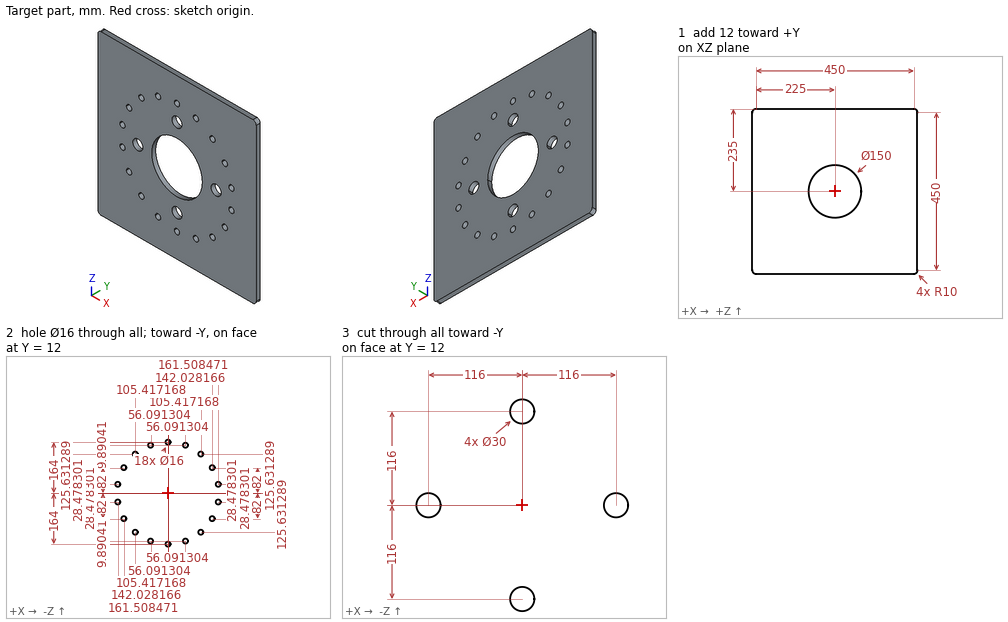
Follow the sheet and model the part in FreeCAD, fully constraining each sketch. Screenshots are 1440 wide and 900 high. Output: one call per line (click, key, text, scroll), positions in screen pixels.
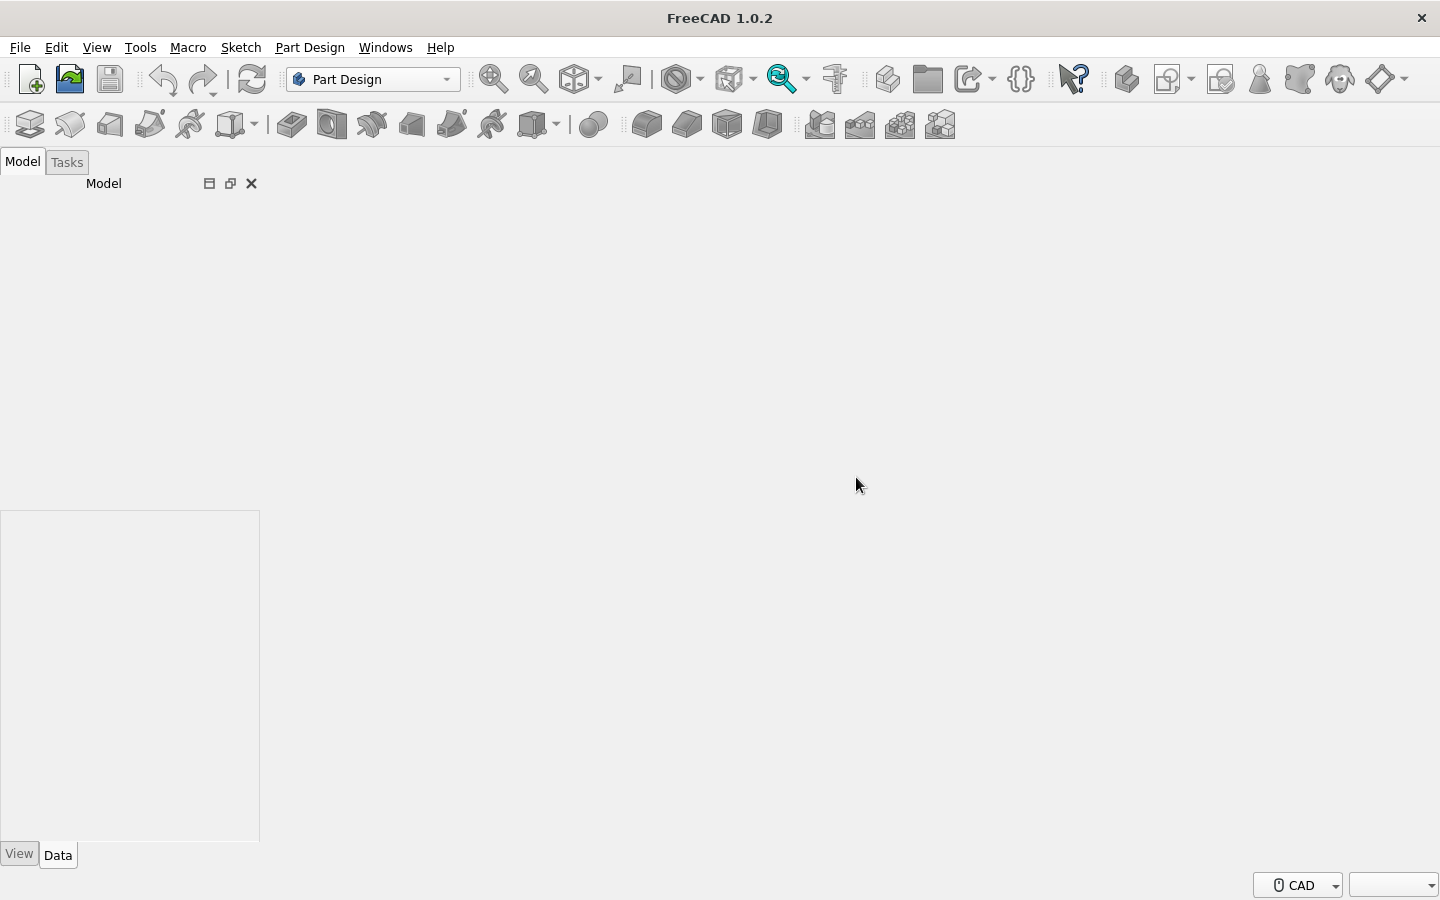
click(30, 80)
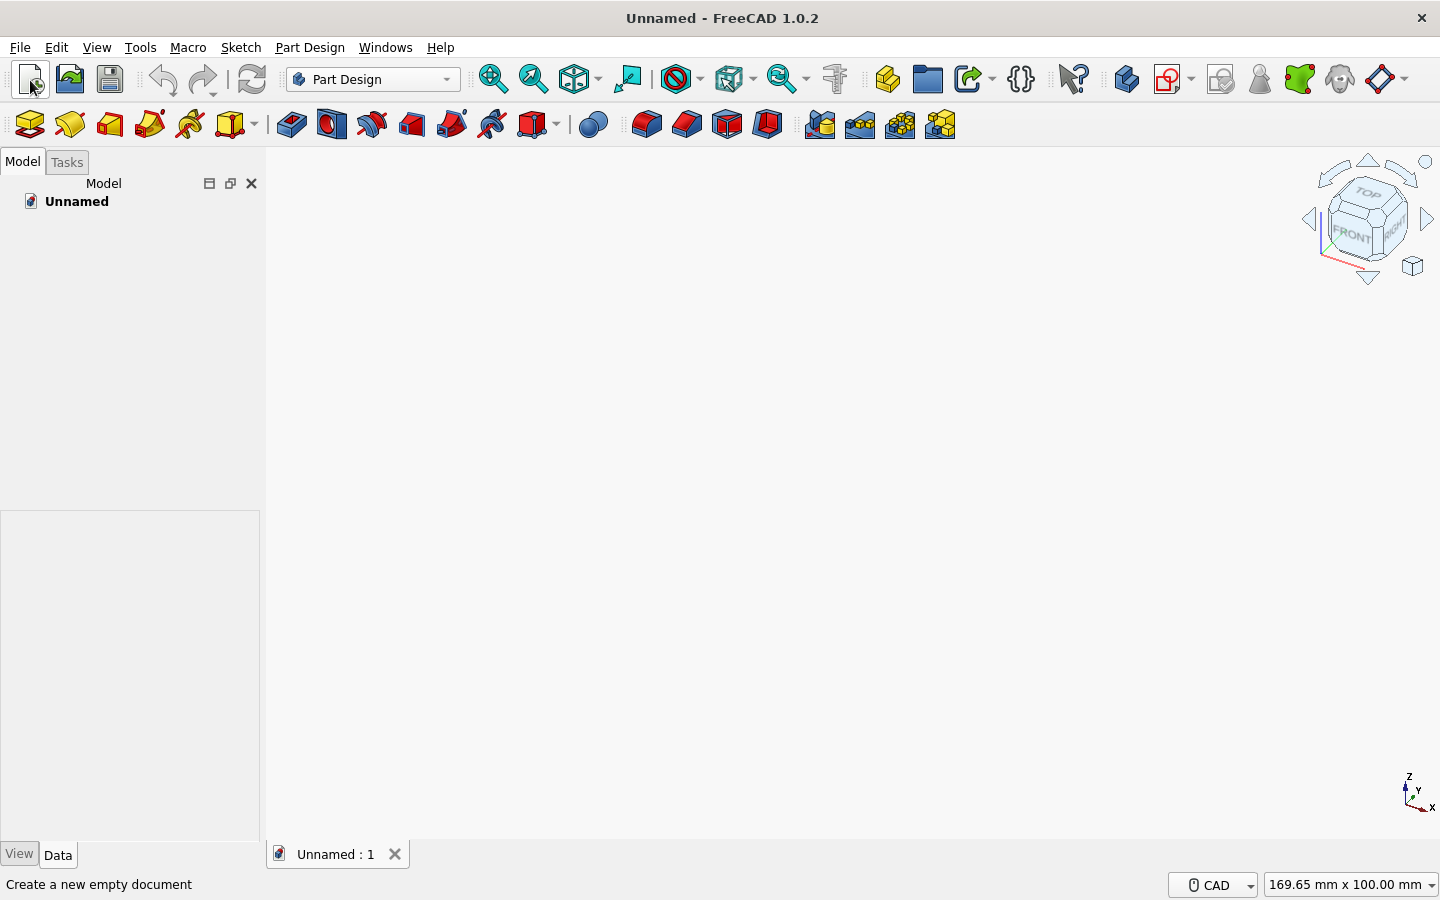
click(1168, 80)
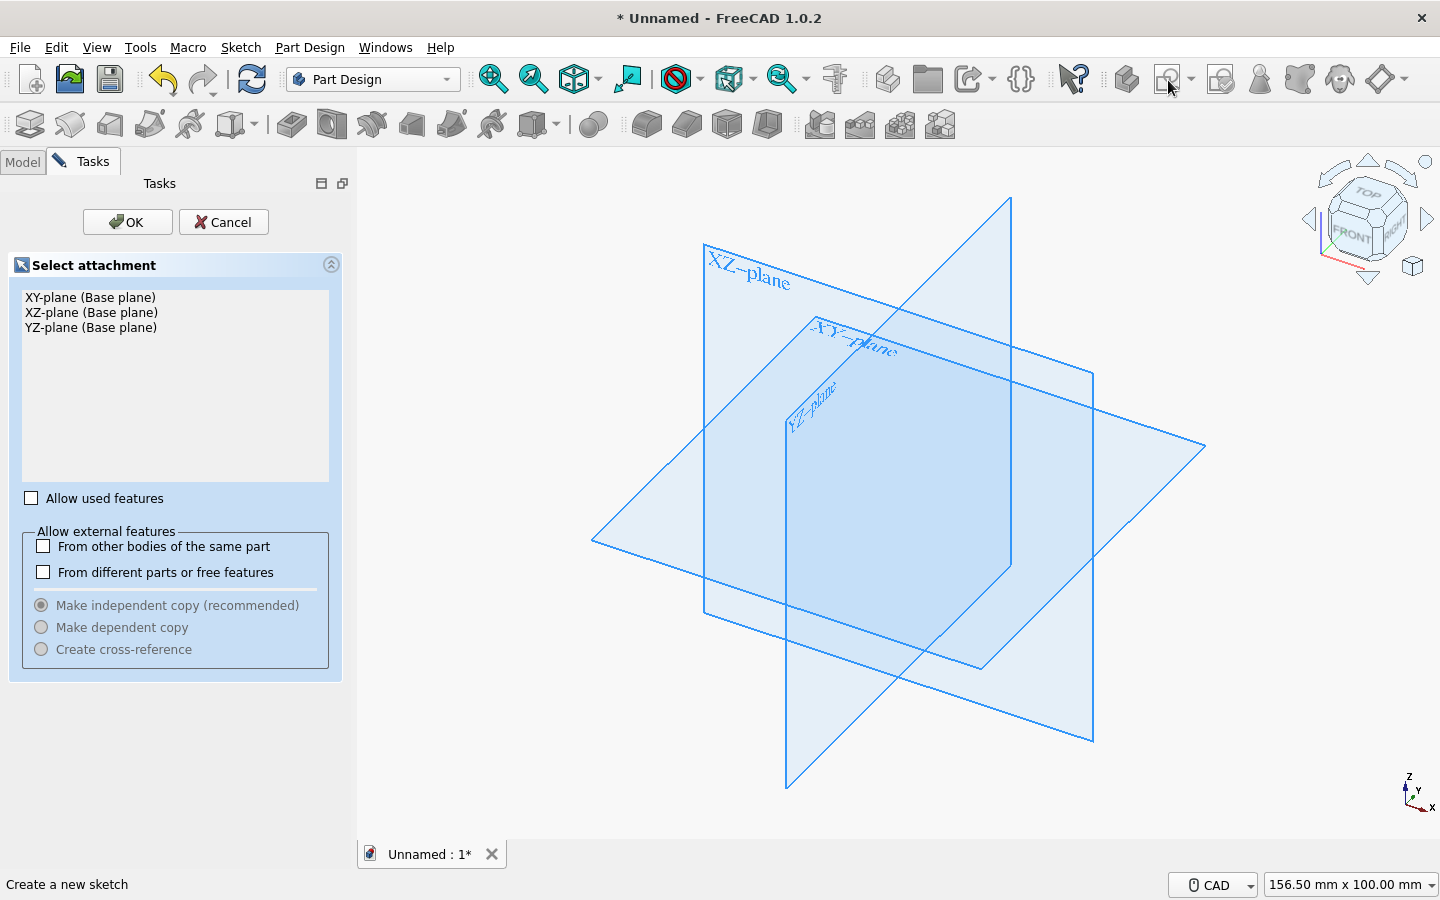
click(82, 312)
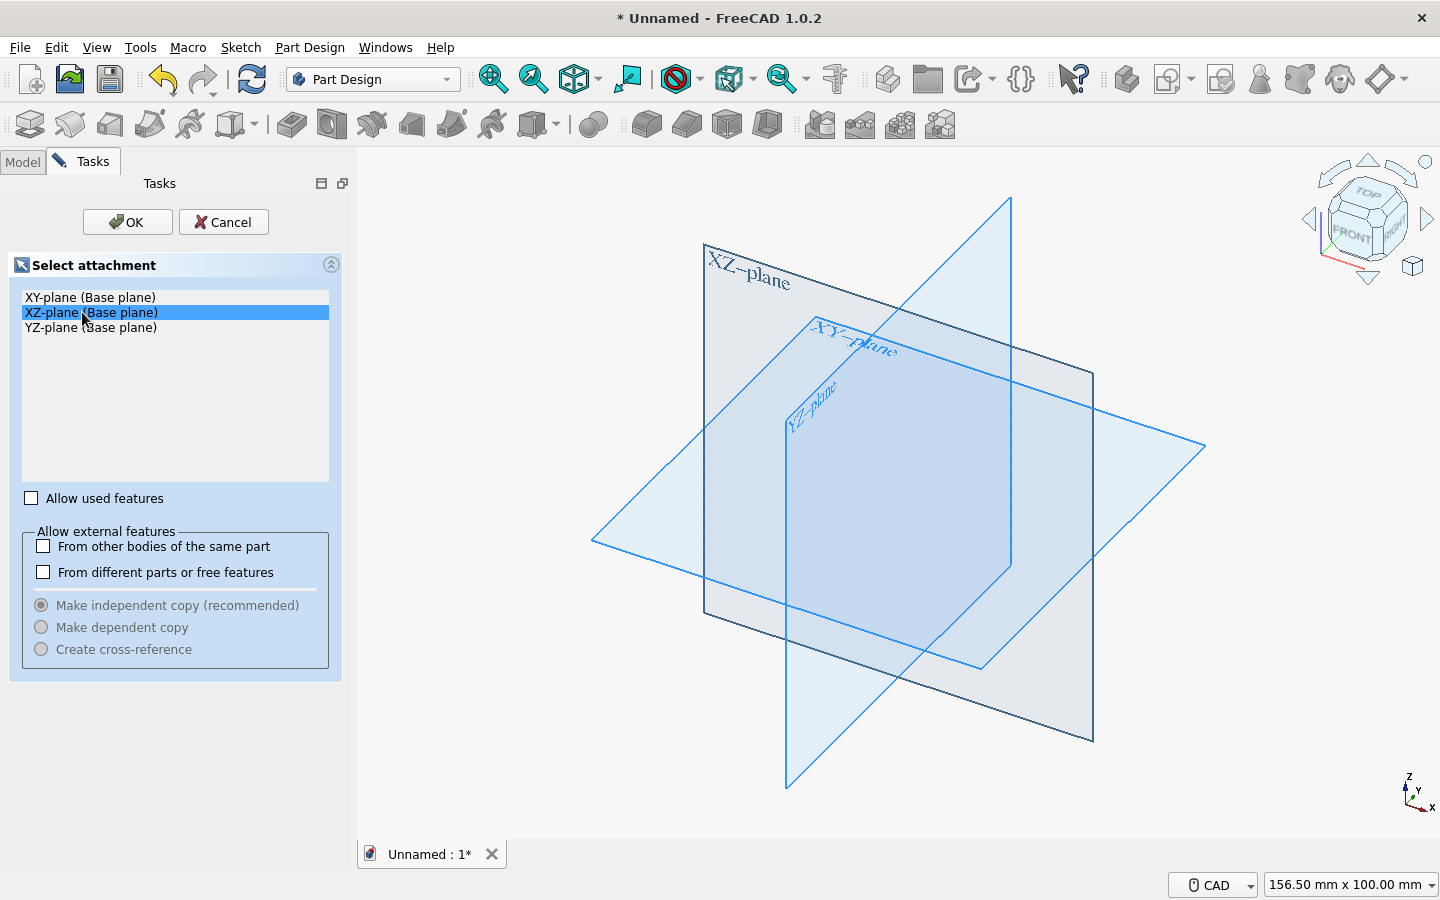
click(128, 222)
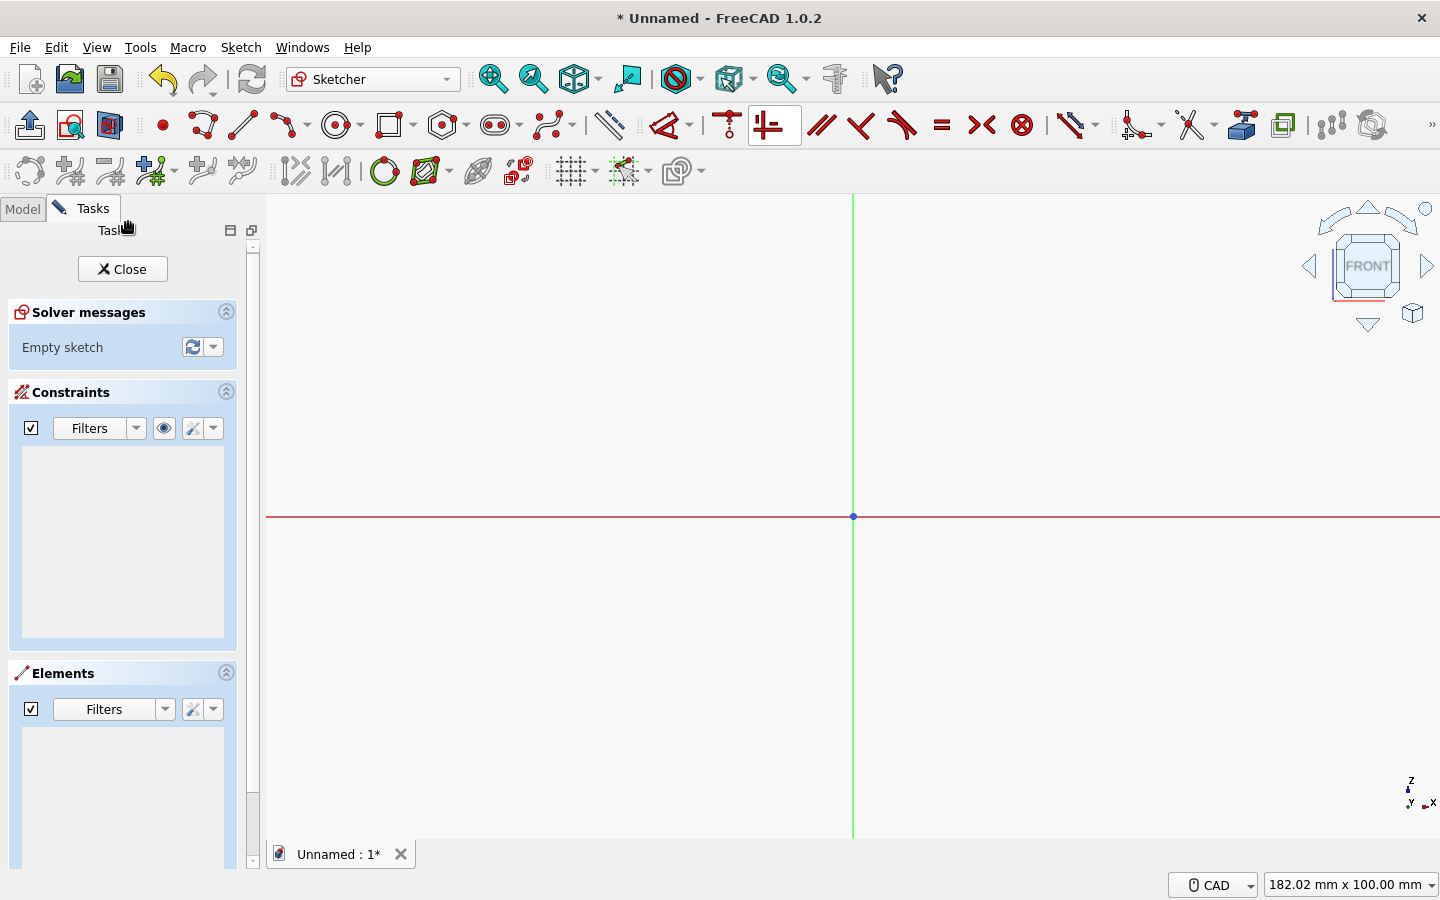
scroll(774, 516, down, 10)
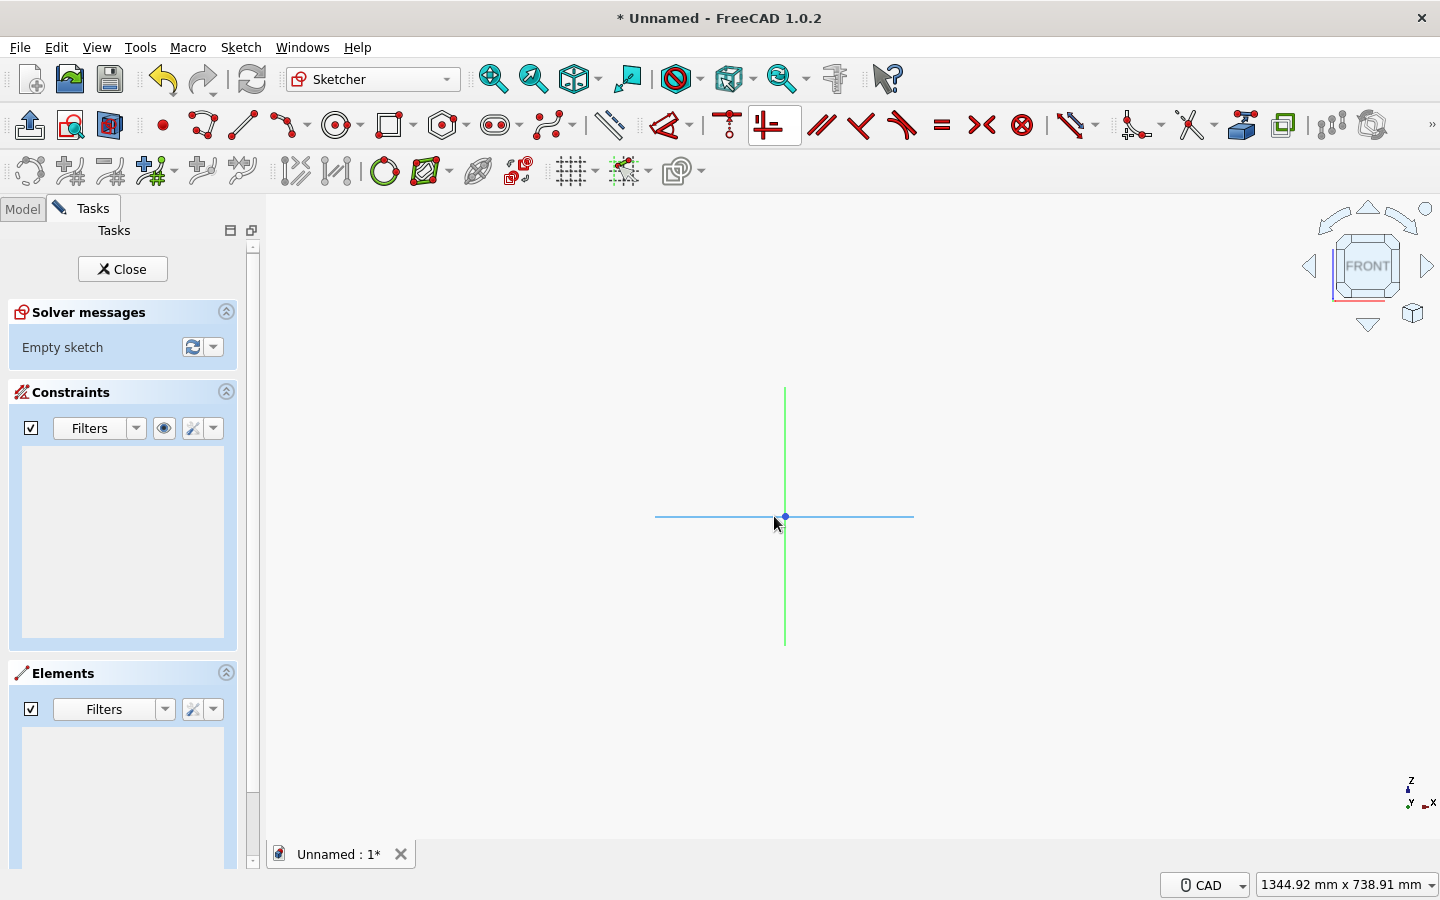
click(244, 126)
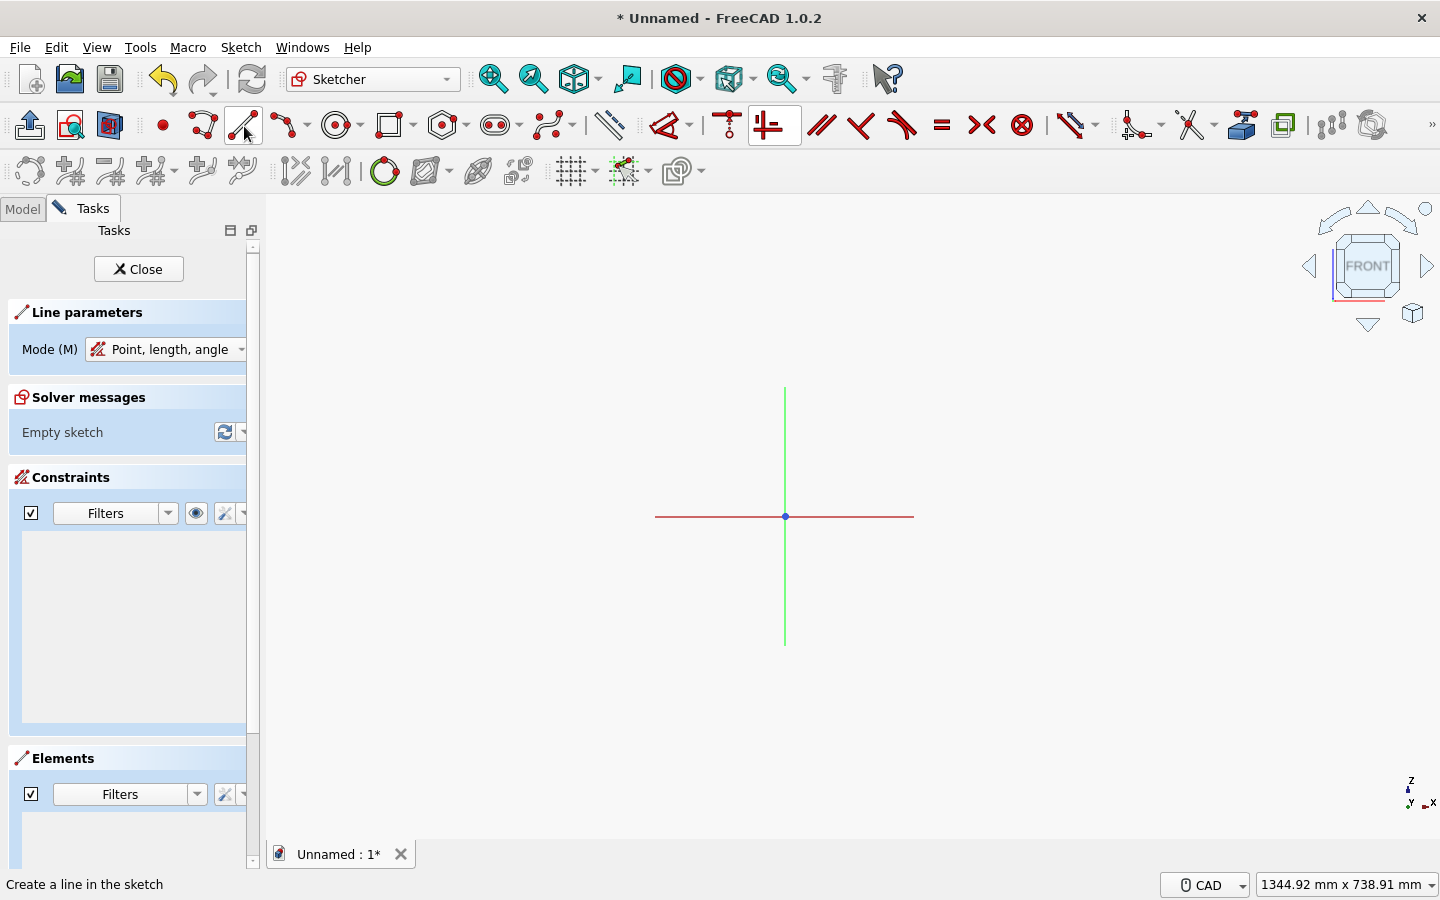
click(589, 311)
click(981, 311)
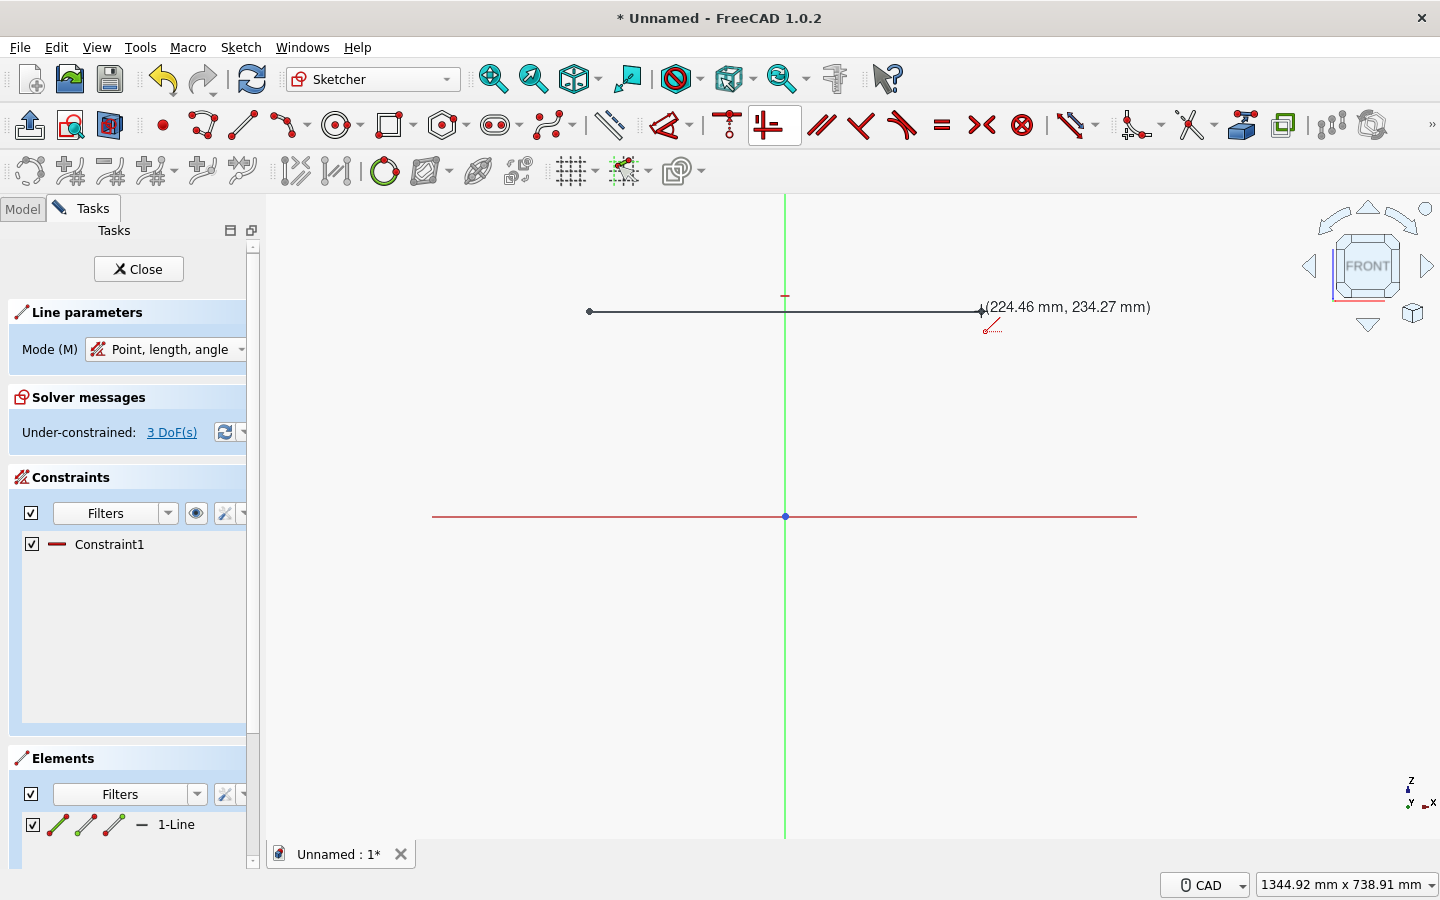
scroll(990, 320, up, 2)